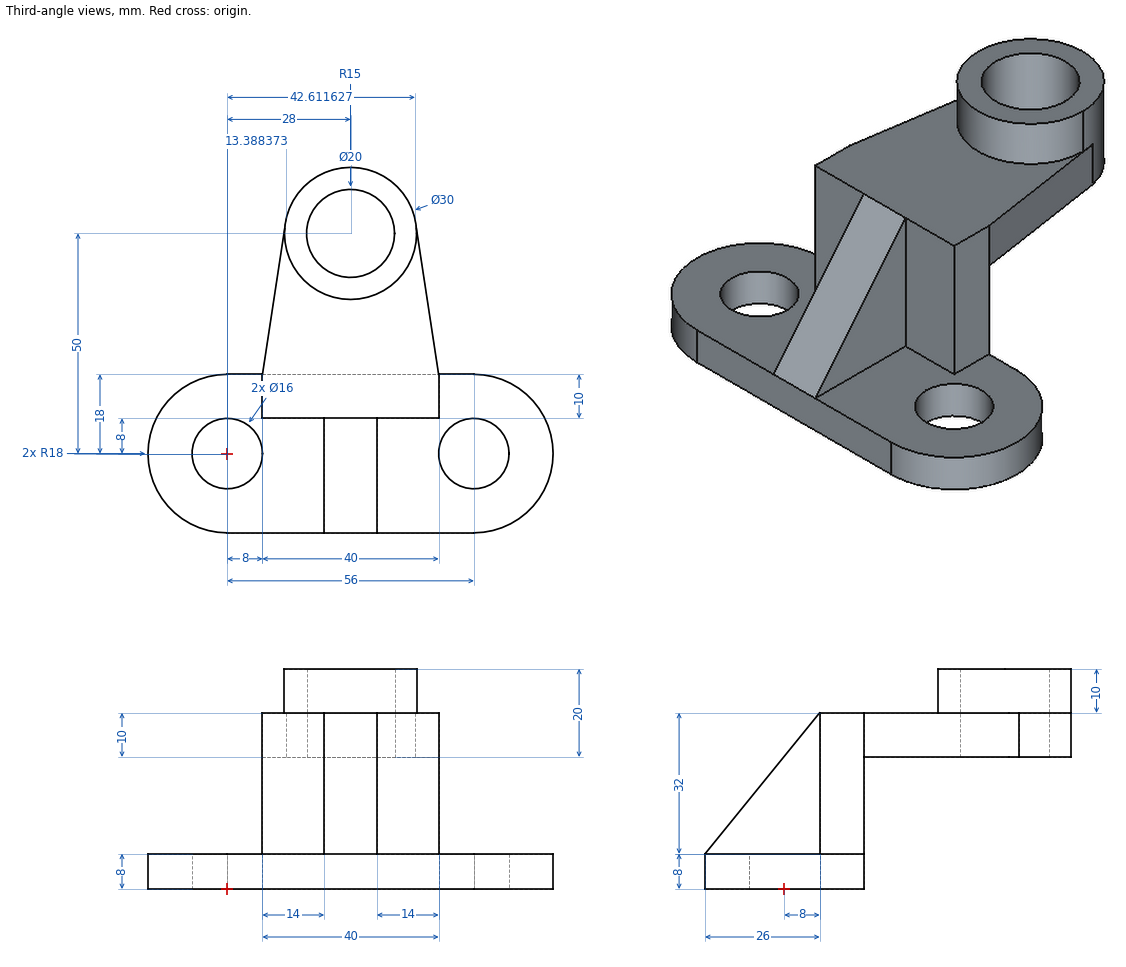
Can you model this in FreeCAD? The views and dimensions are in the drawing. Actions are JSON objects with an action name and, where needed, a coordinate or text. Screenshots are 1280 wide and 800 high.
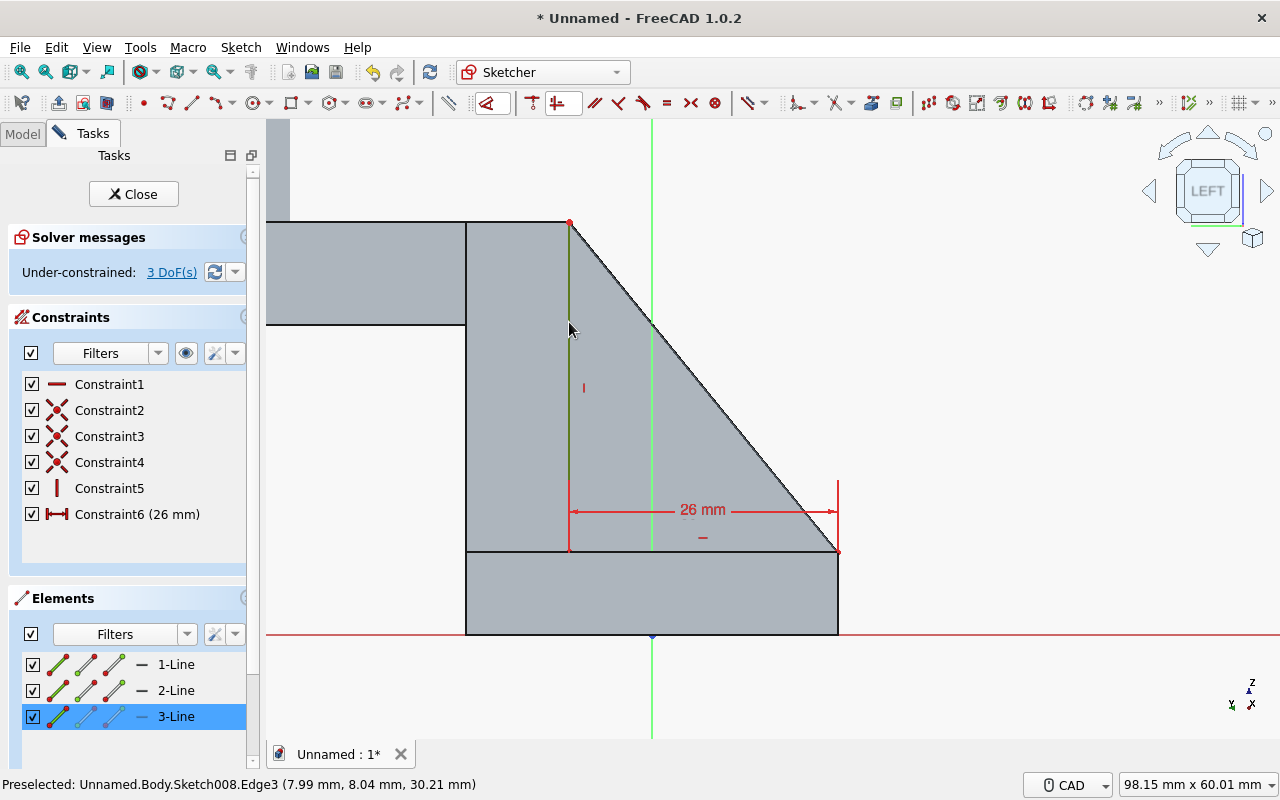
{"action": "left_click", "coordinate": [504, 104]}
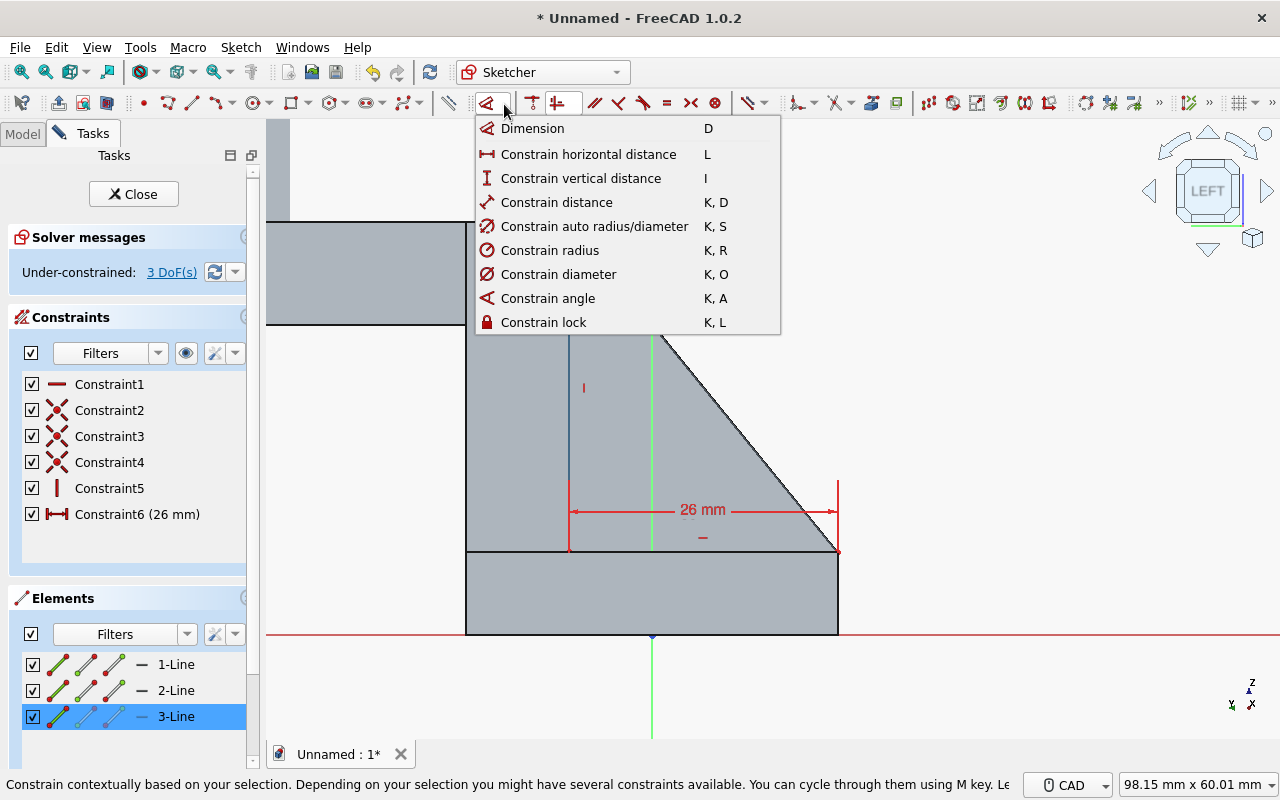
{"action": "left_click", "coordinate": [628, 178]}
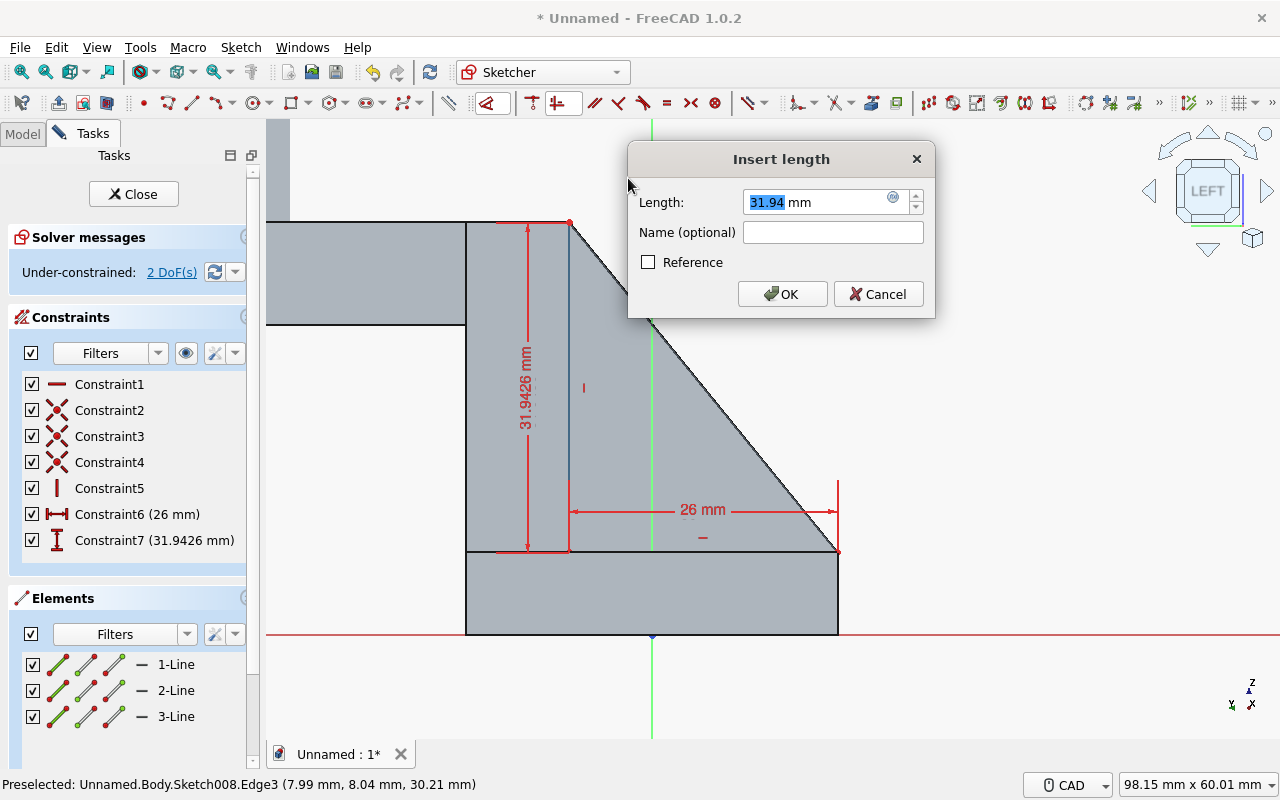
{"action": "type", "text": "32"}
{"action": "key", "text": "Return"}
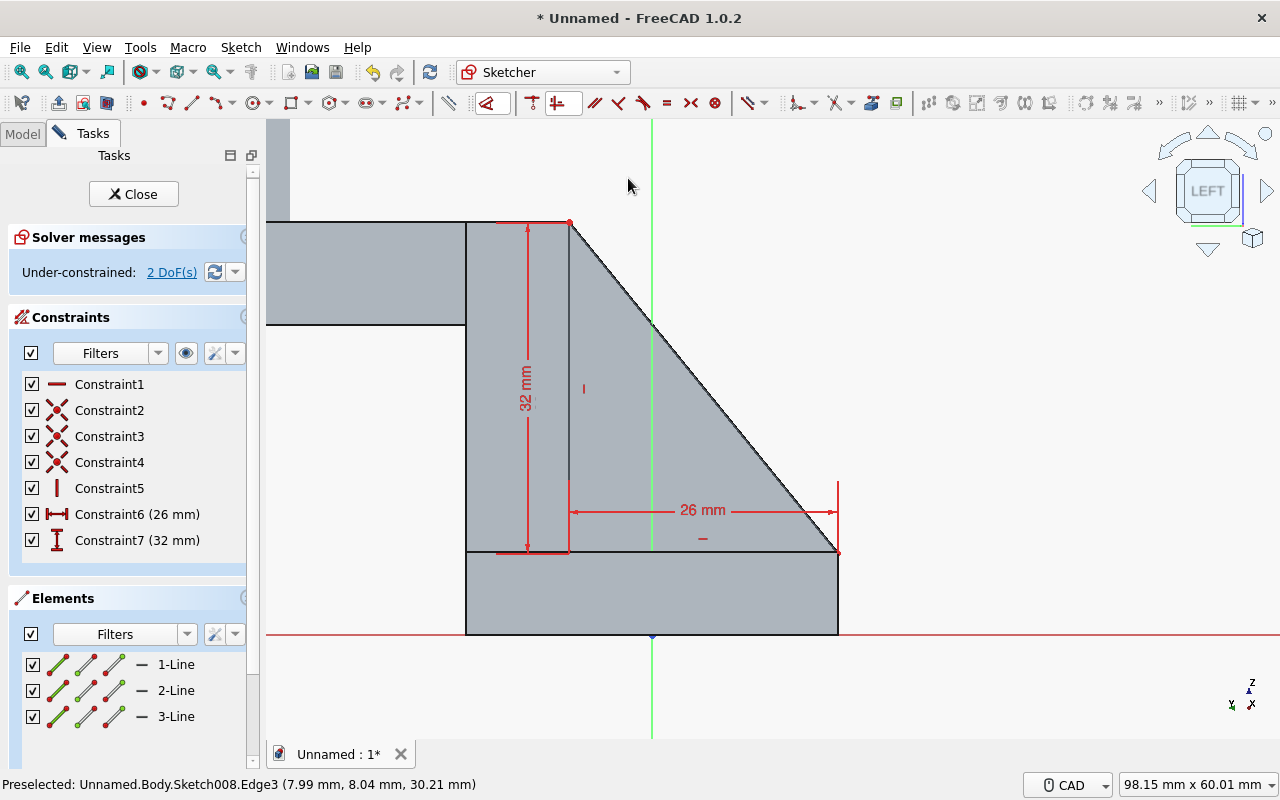
{"action": "left_click", "coordinate": [569, 554]}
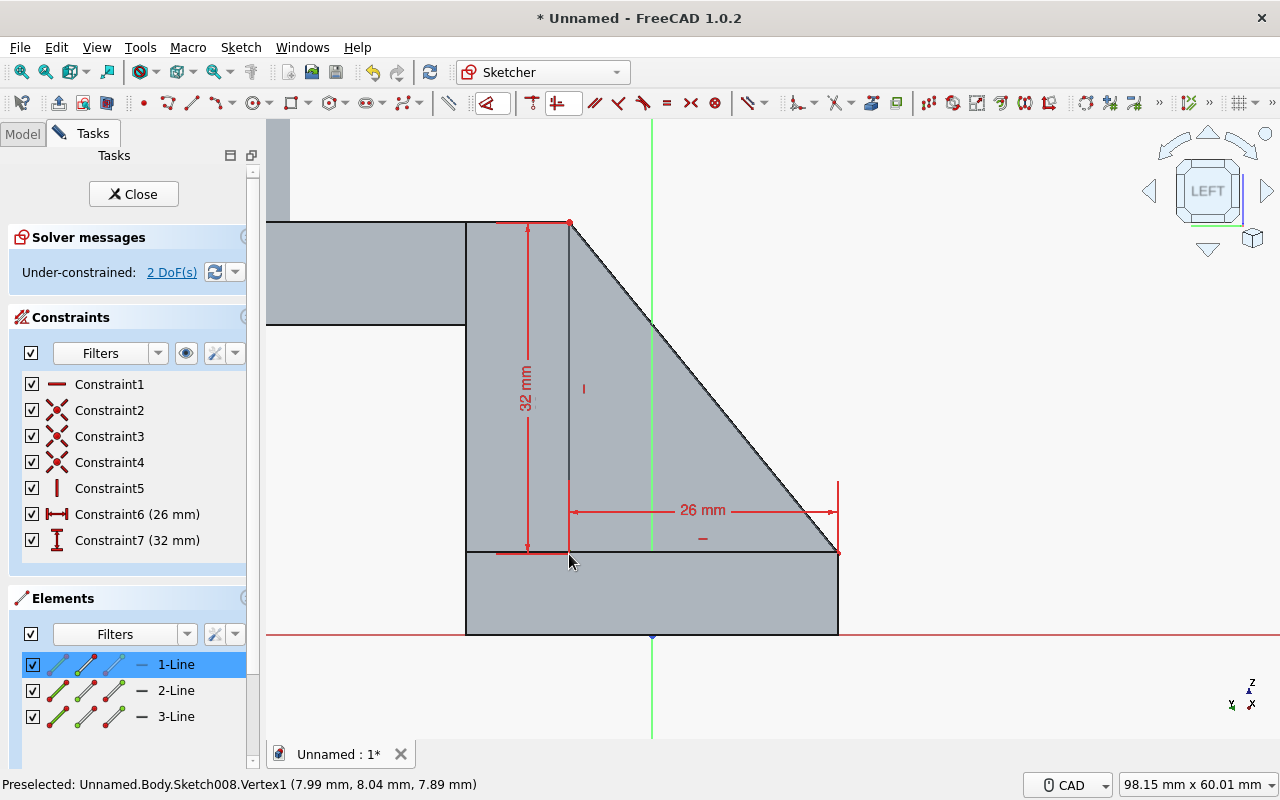
{"action": "key", "text": "l"}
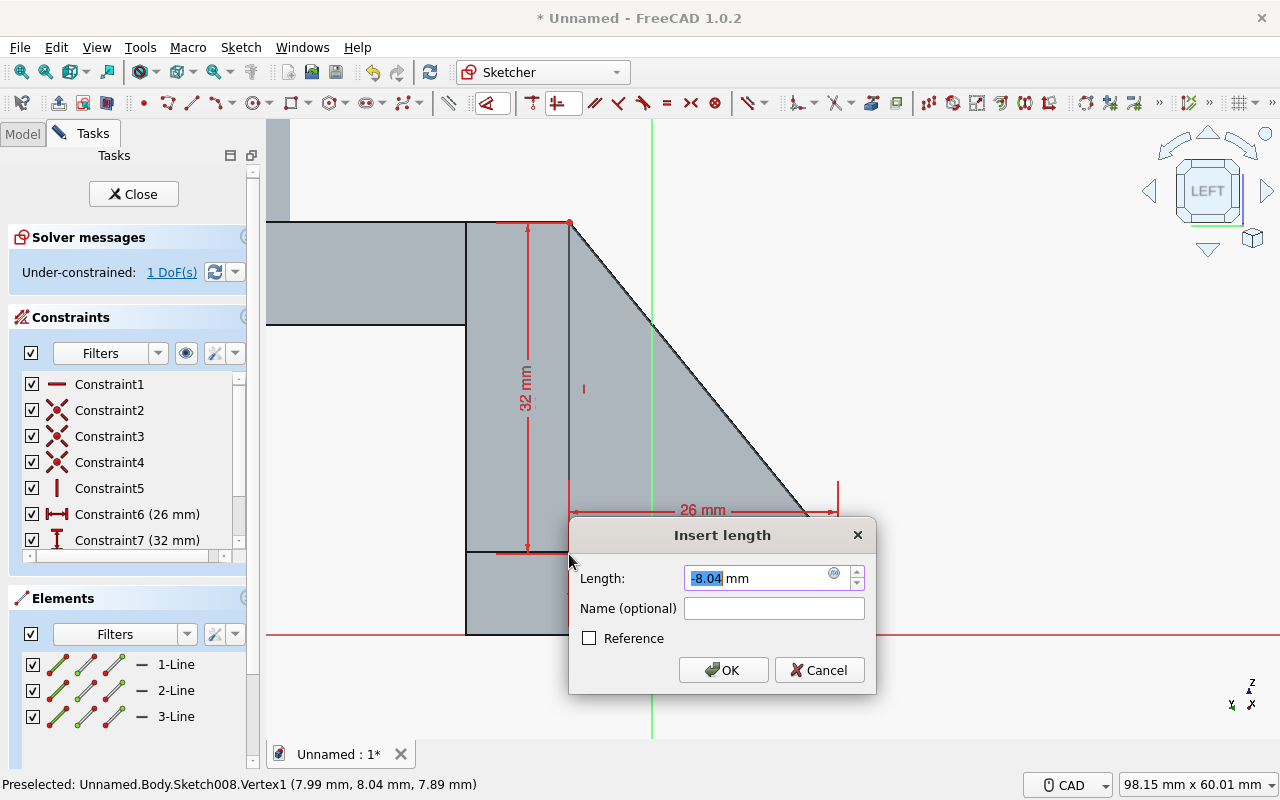
{"action": "type", "text": "-8"}
{"action": "key", "text": "Return"}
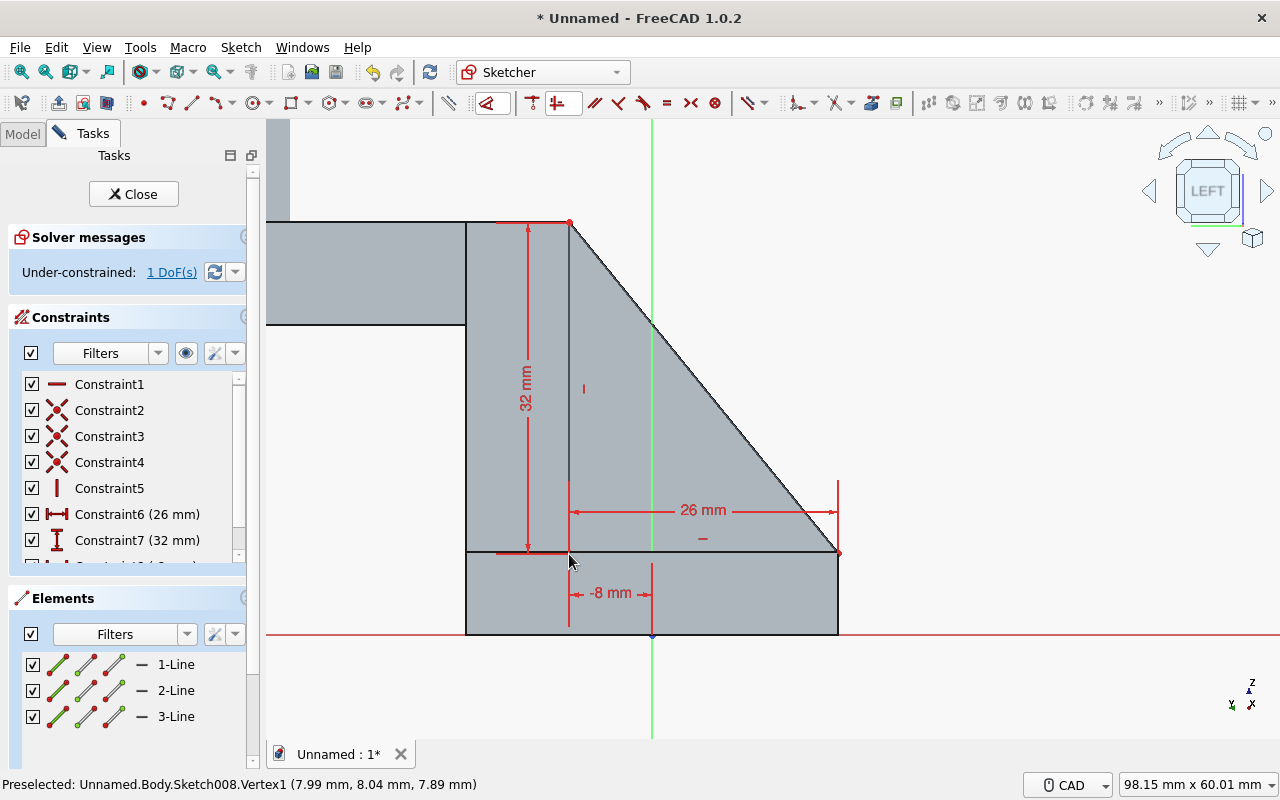
{"action": "left_click", "coordinate": [569, 554]}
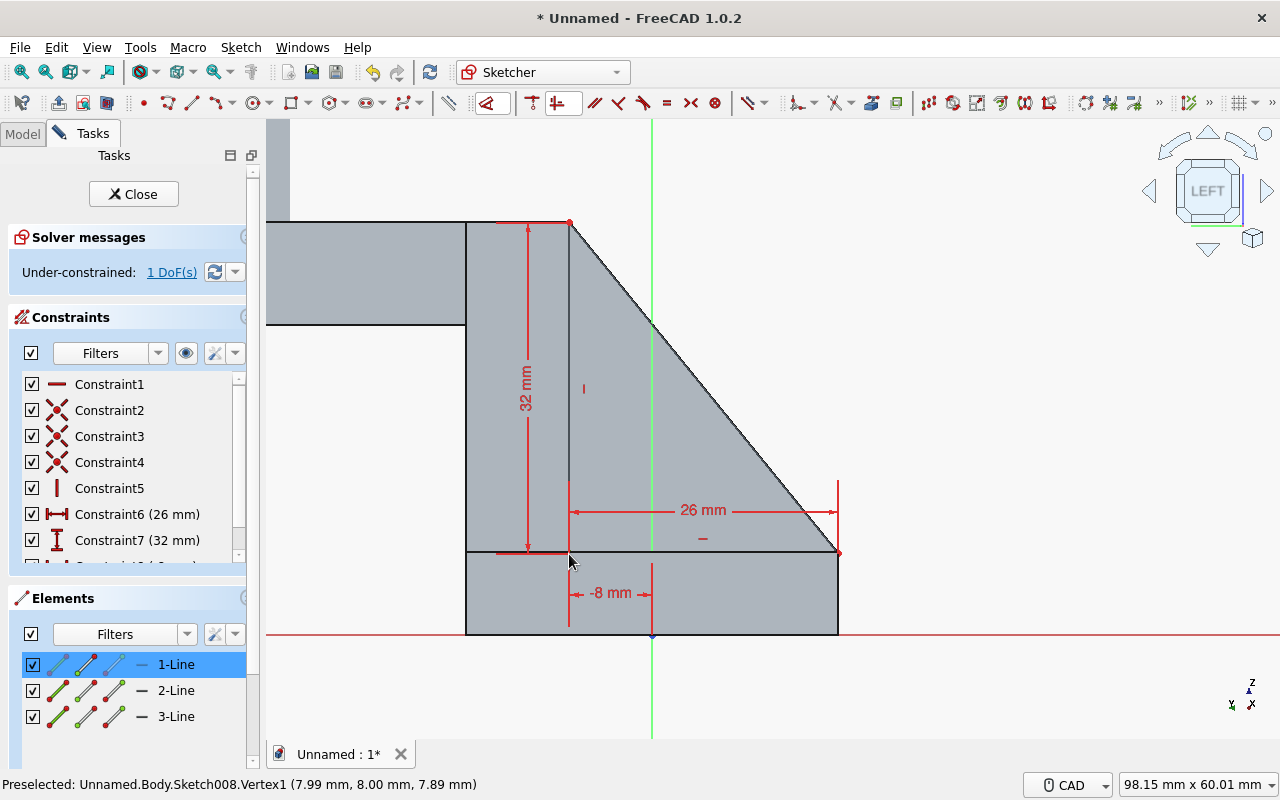
{"action": "left_click", "coordinate": [504, 104]}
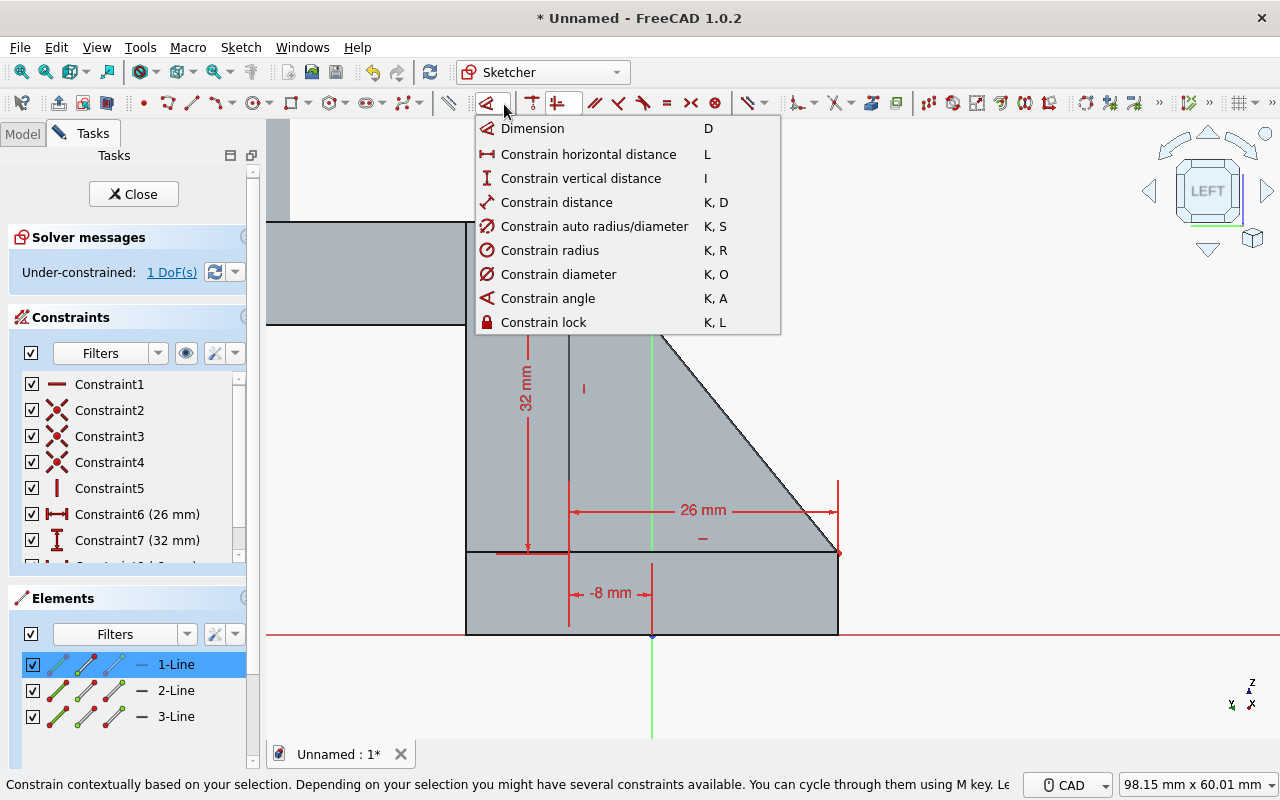
{"action": "left_click", "coordinate": [628, 178]}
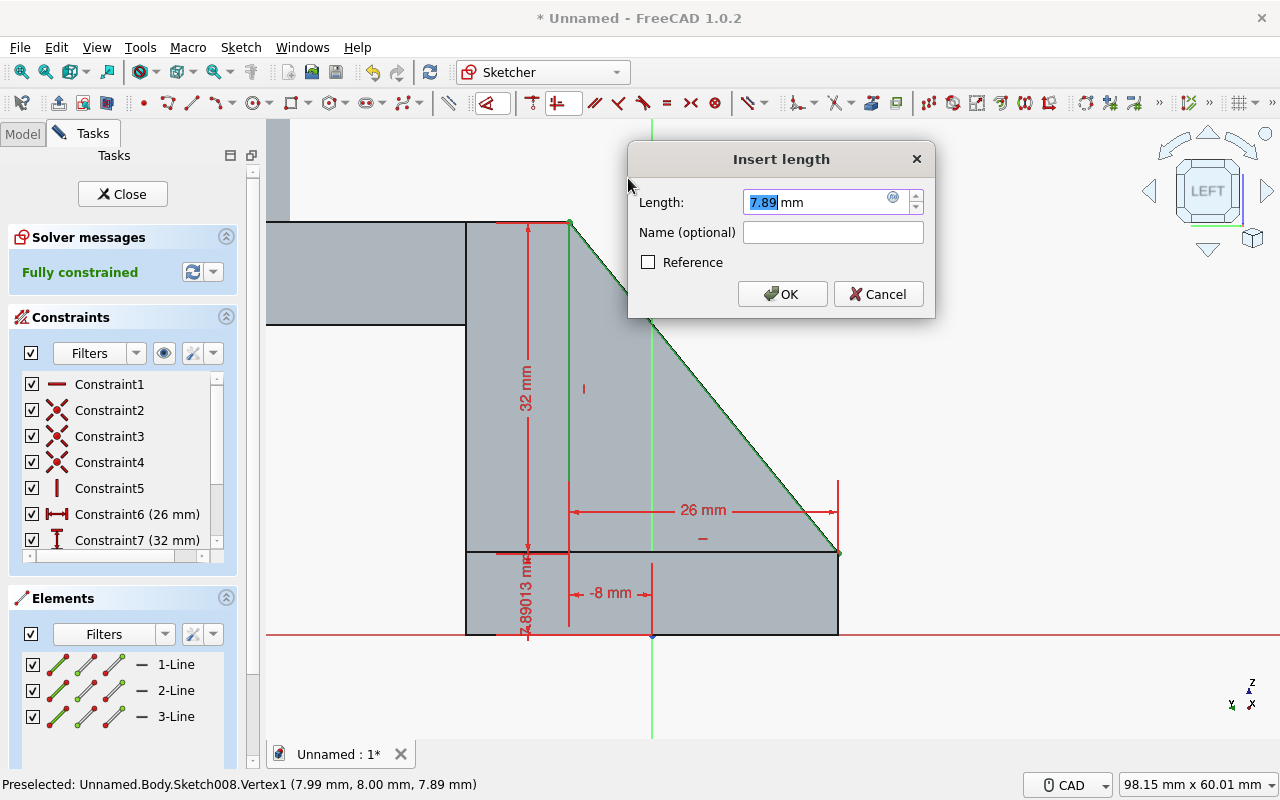
{"action": "type", "text": "8"}
{"action": "key", "text": "Return"}